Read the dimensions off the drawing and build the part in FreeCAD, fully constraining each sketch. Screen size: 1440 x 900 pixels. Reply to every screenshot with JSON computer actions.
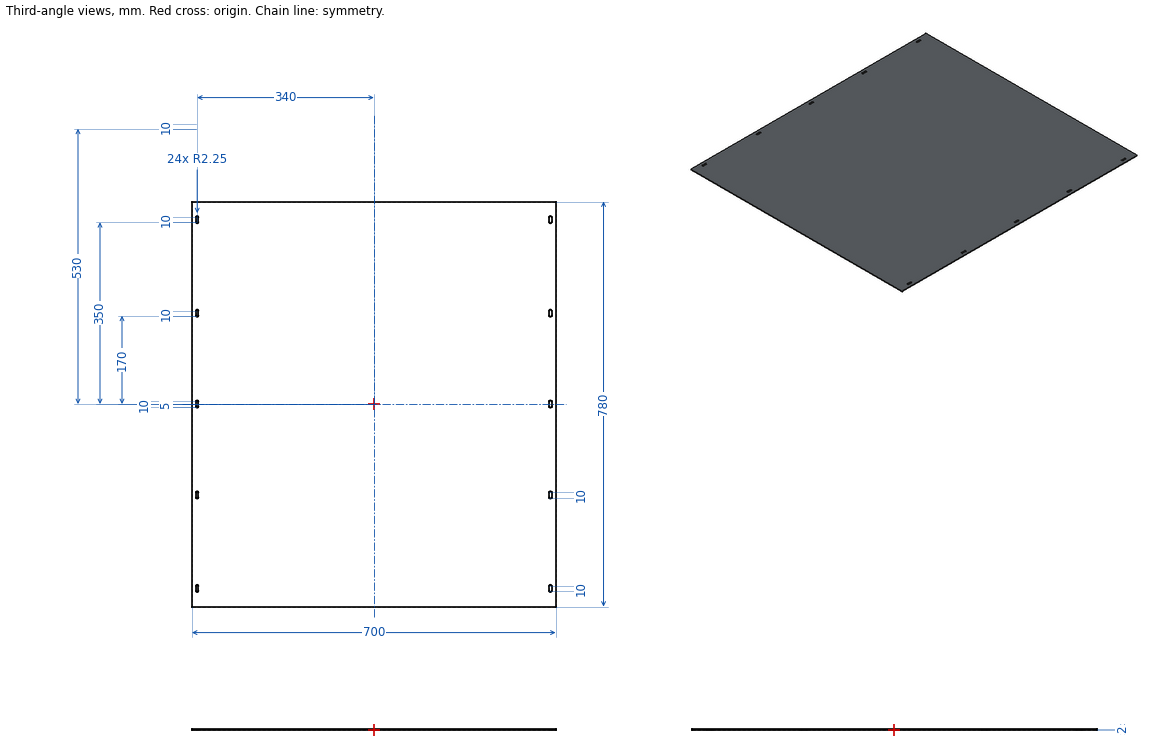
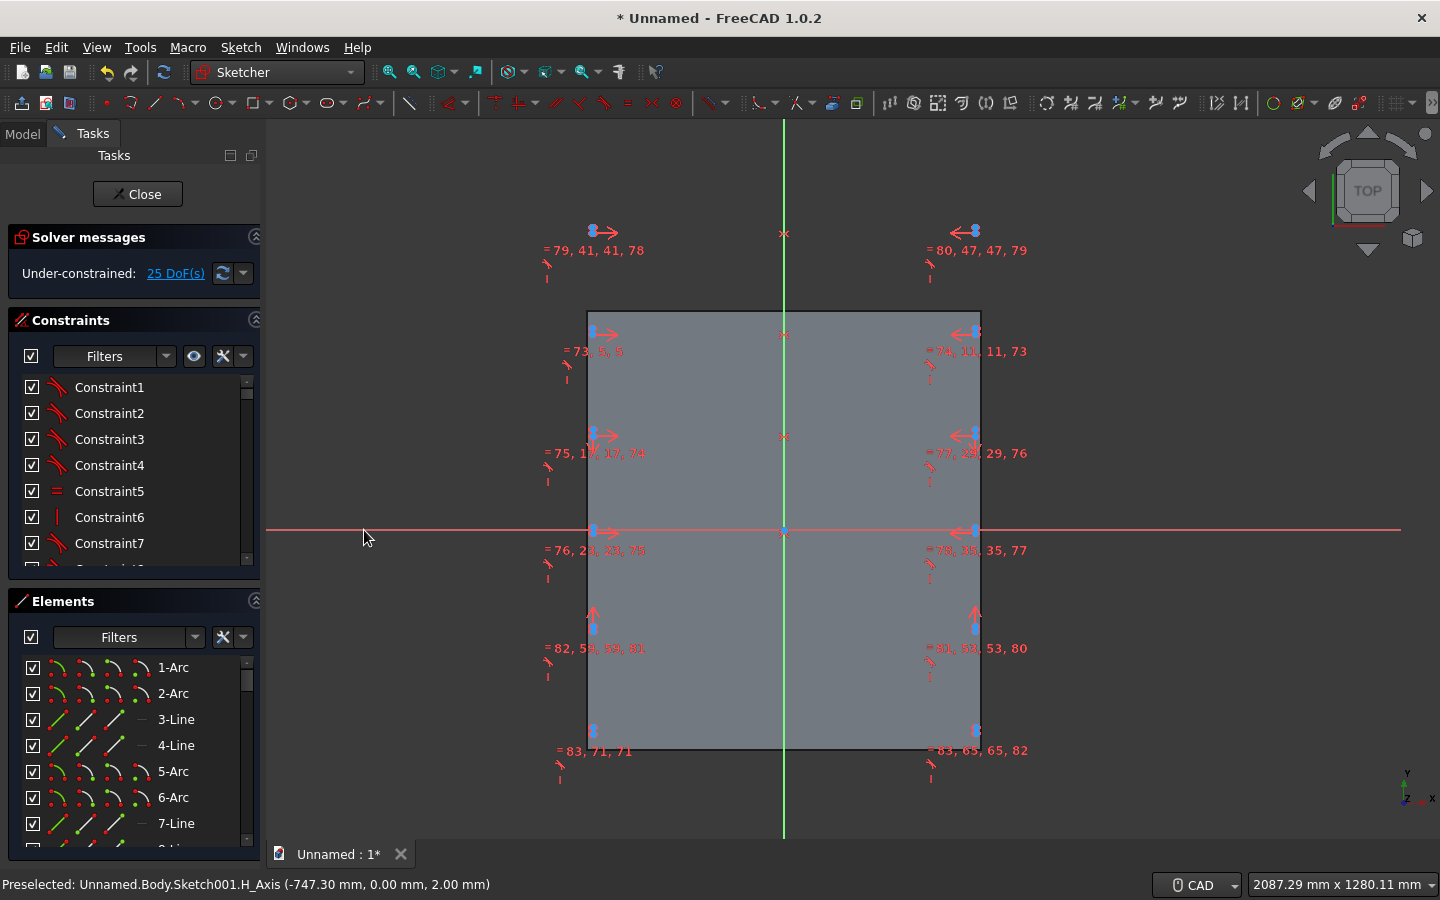
{"action": "scroll", "coordinate": [976, 328], "scroll_direction": "up", "scroll_amount": 12}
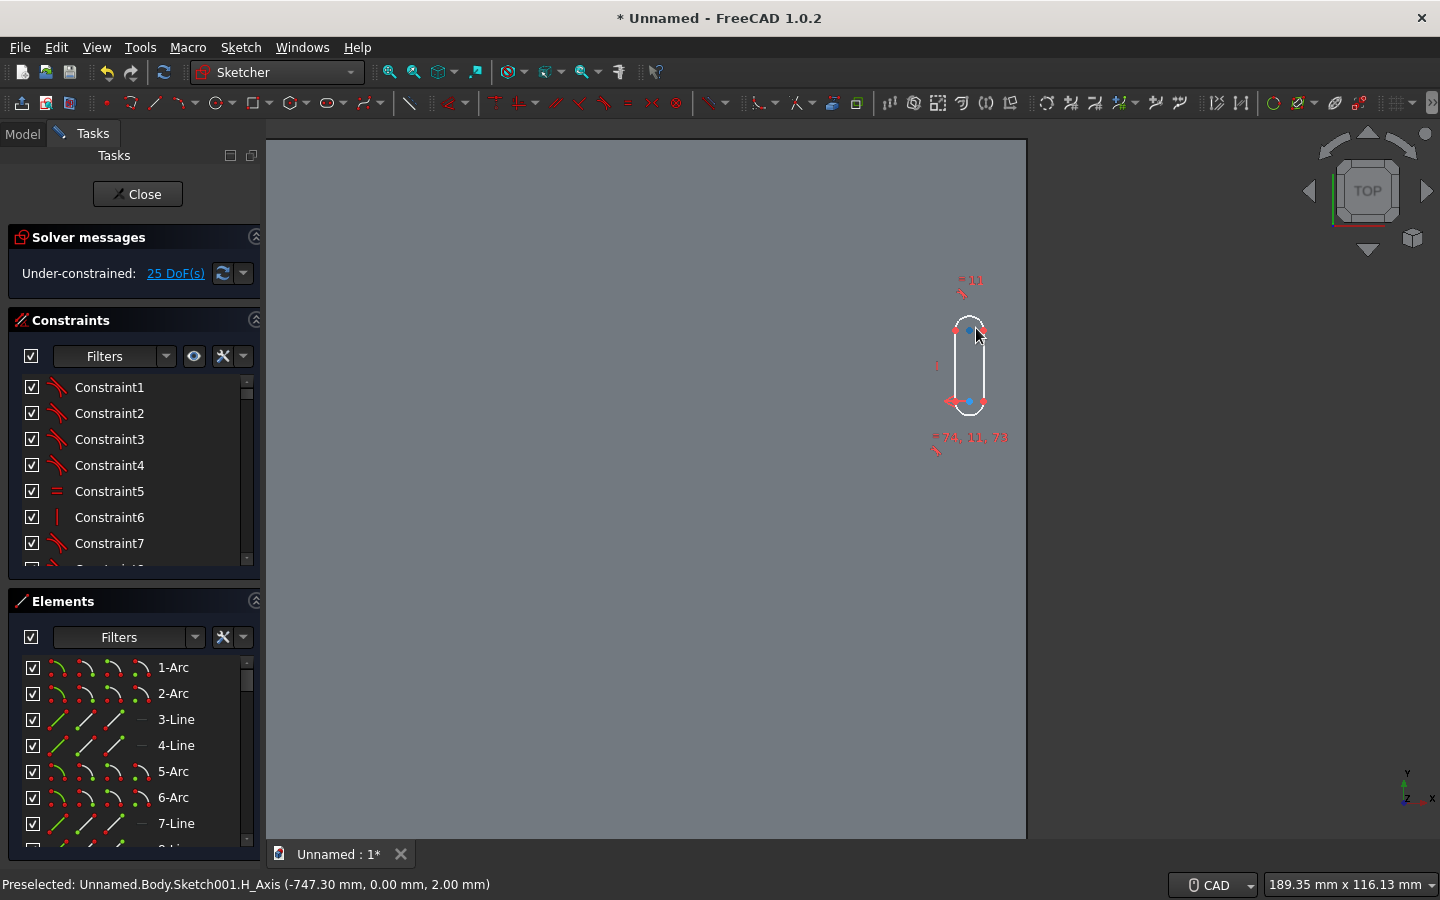
{"action": "left_click", "coordinate": [970, 330]}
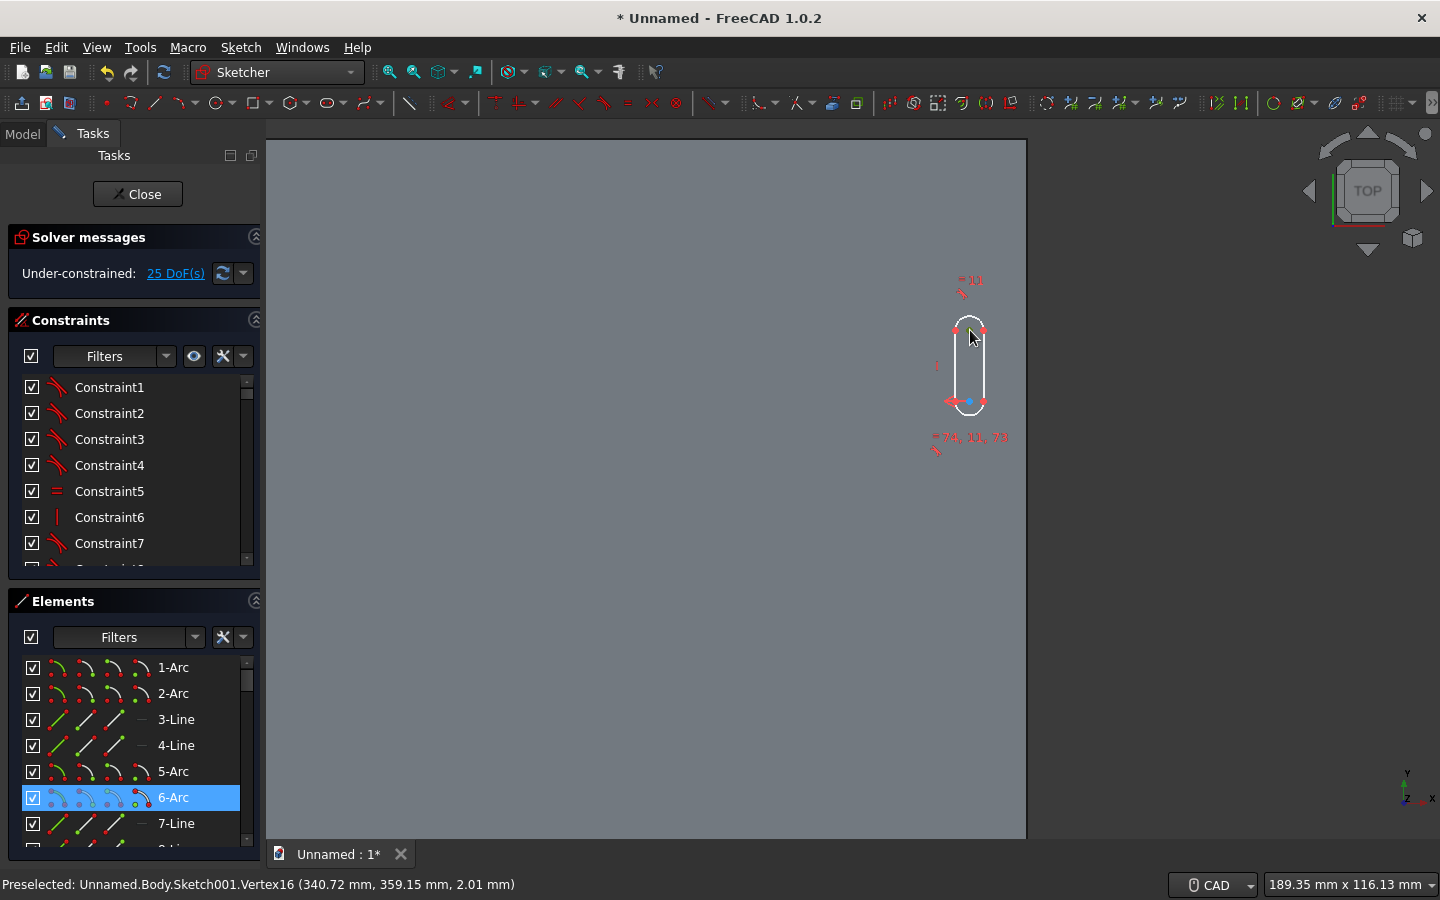
{"action": "scroll", "coordinate": [977, 327], "scroll_direction": "down", "scroll_amount": 12}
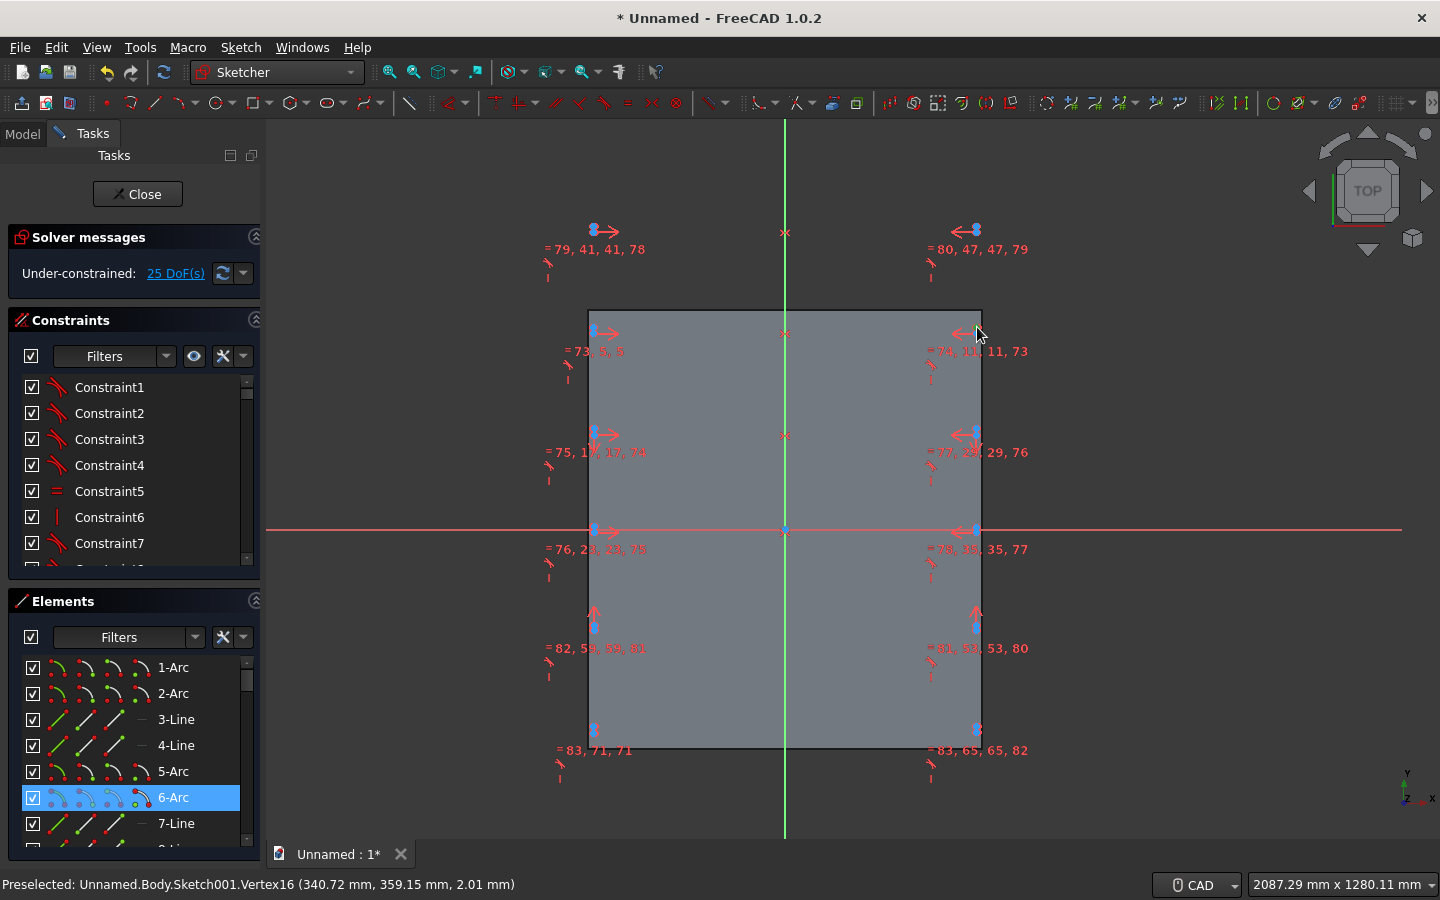
{"action": "scroll", "coordinate": [977, 733], "scroll_direction": "up", "scroll_amount": 12}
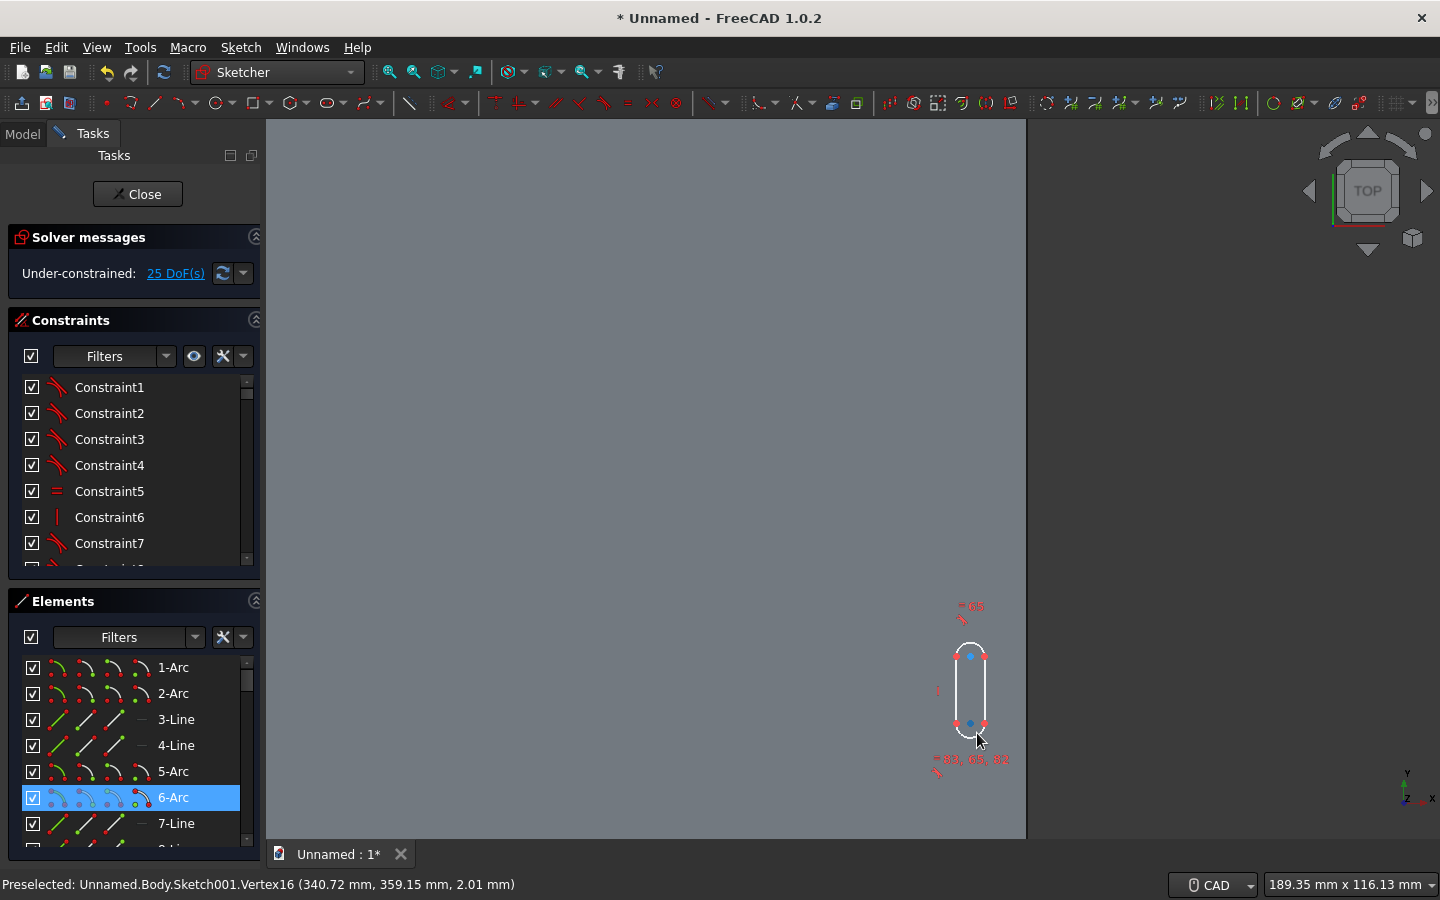
{"action": "left_click", "coordinate": [970, 724]}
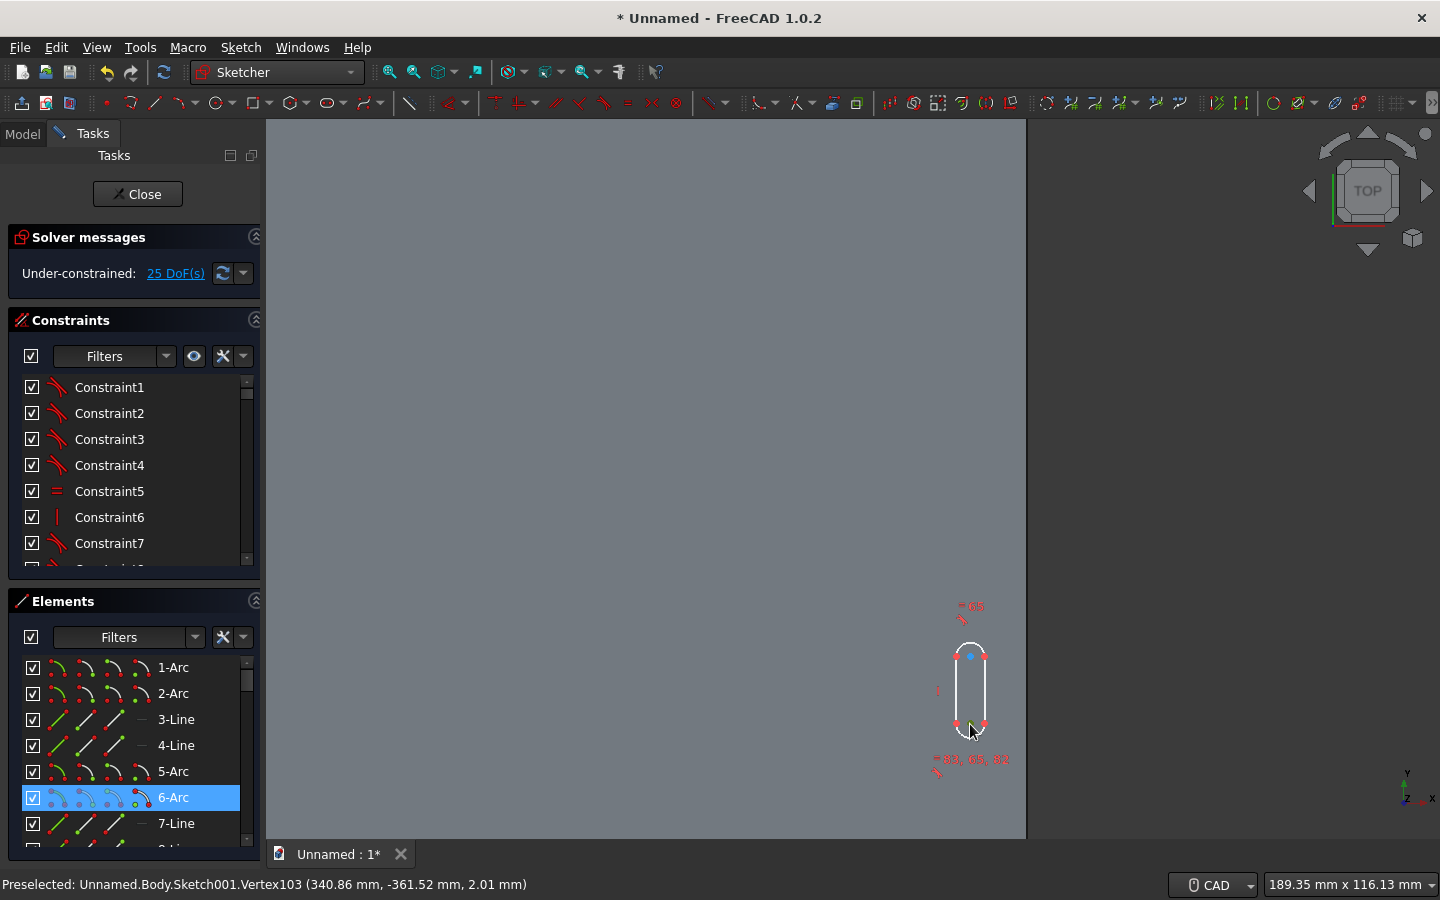
{"action": "scroll", "coordinate": [977, 734], "scroll_direction": "down", "scroll_amount": 12}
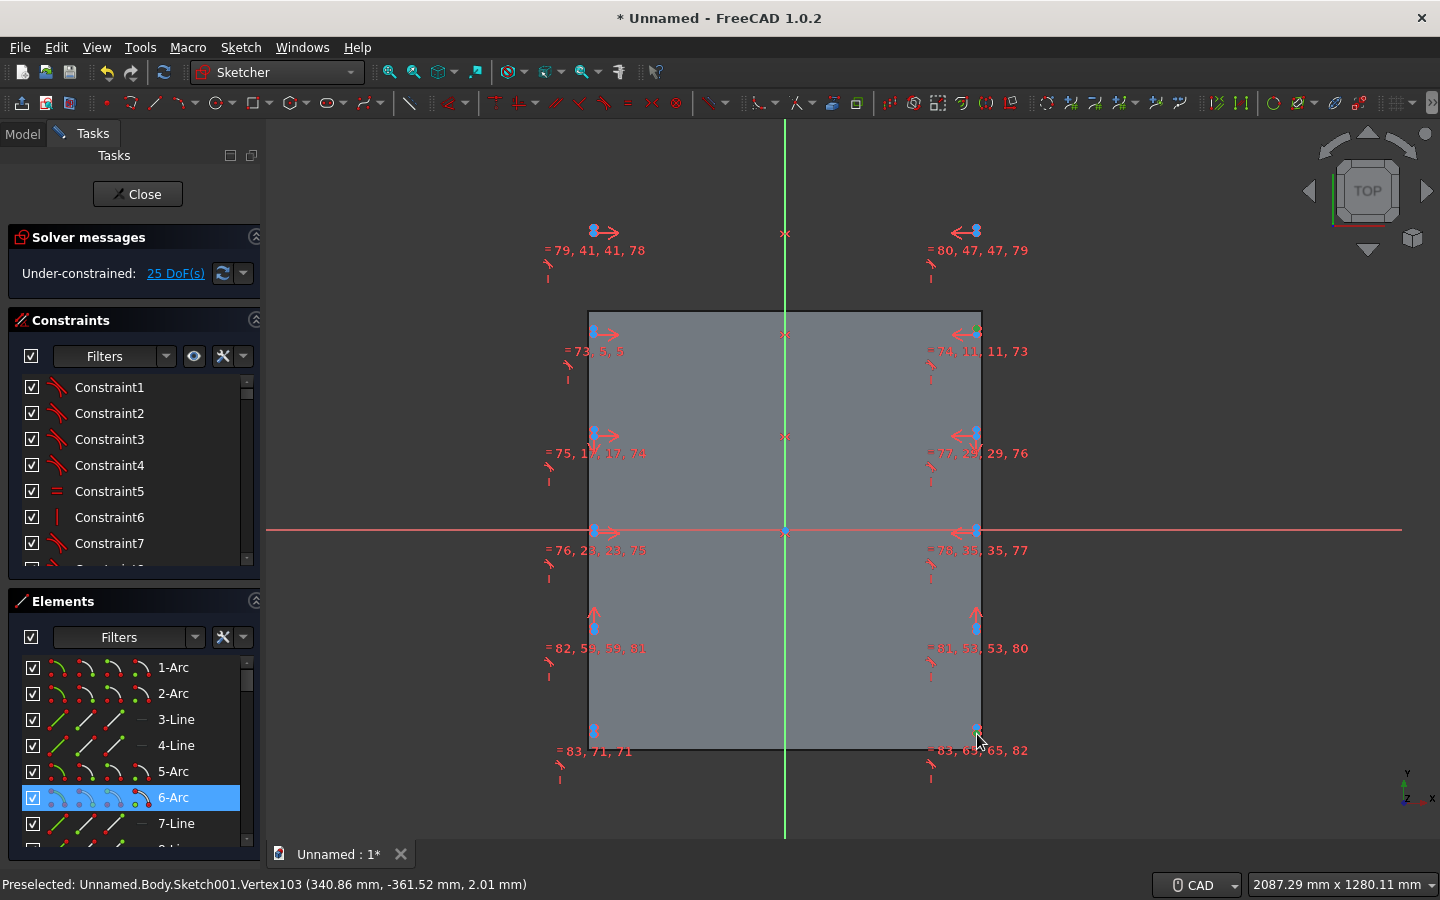
{"action": "left_click", "coordinate": [364, 530]}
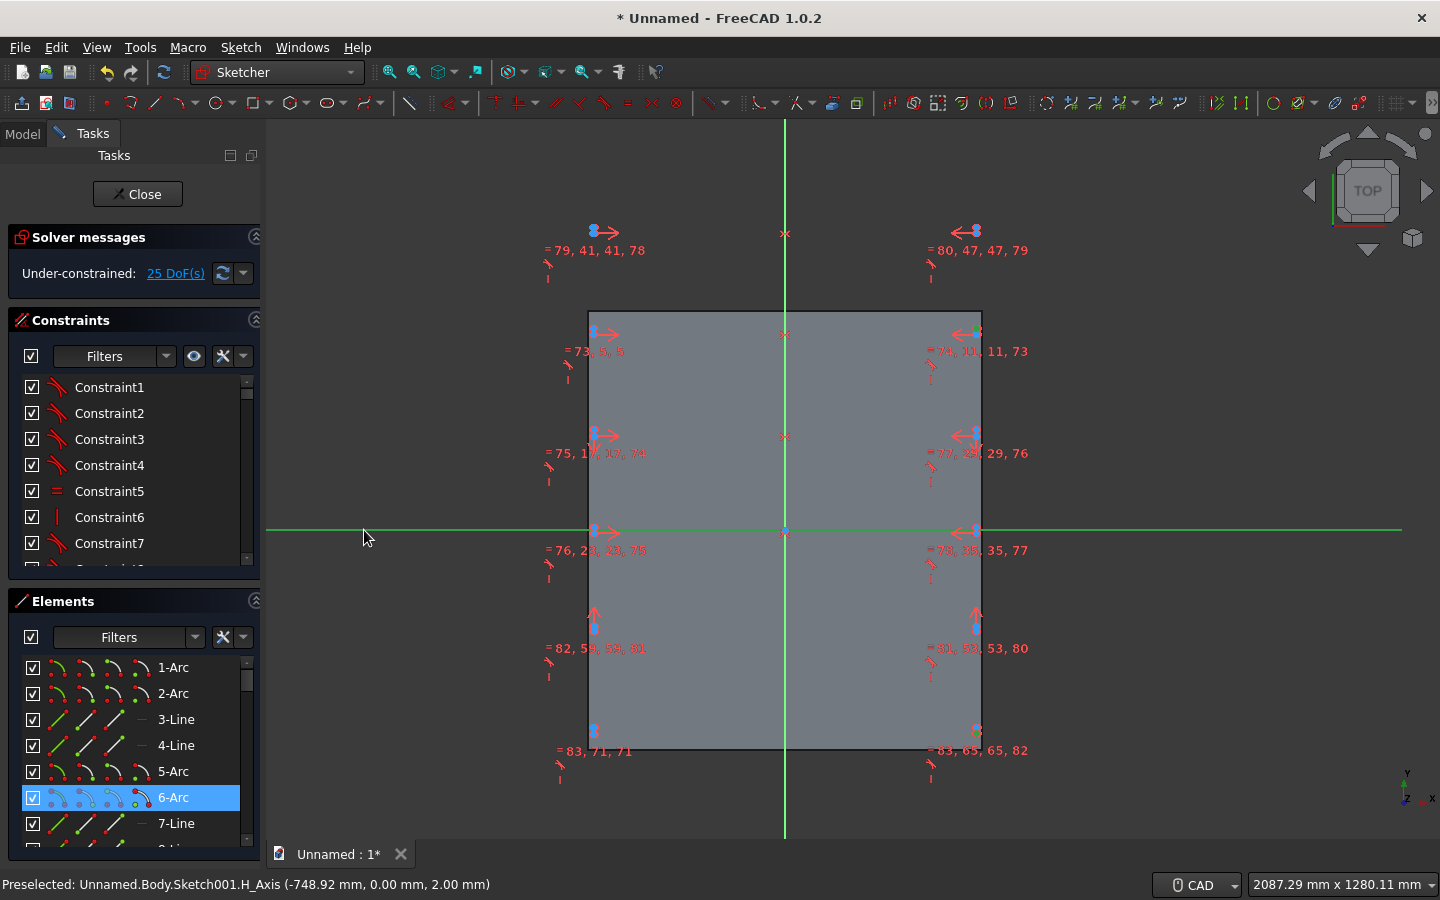
{"action": "key", "text": "s"}